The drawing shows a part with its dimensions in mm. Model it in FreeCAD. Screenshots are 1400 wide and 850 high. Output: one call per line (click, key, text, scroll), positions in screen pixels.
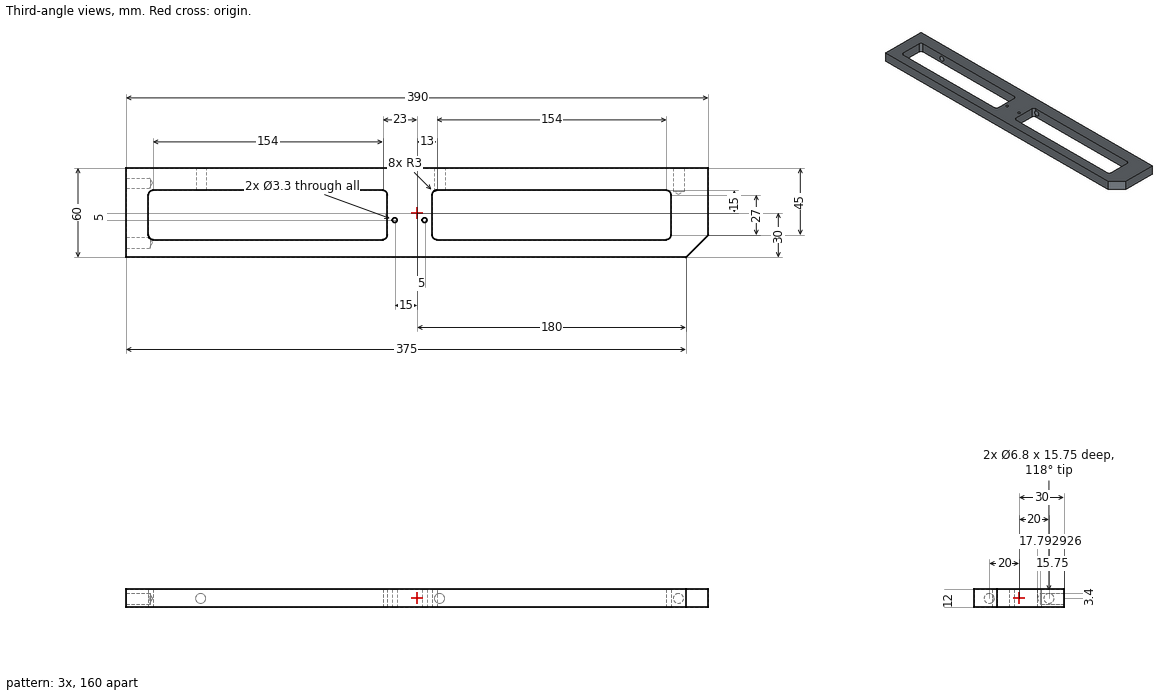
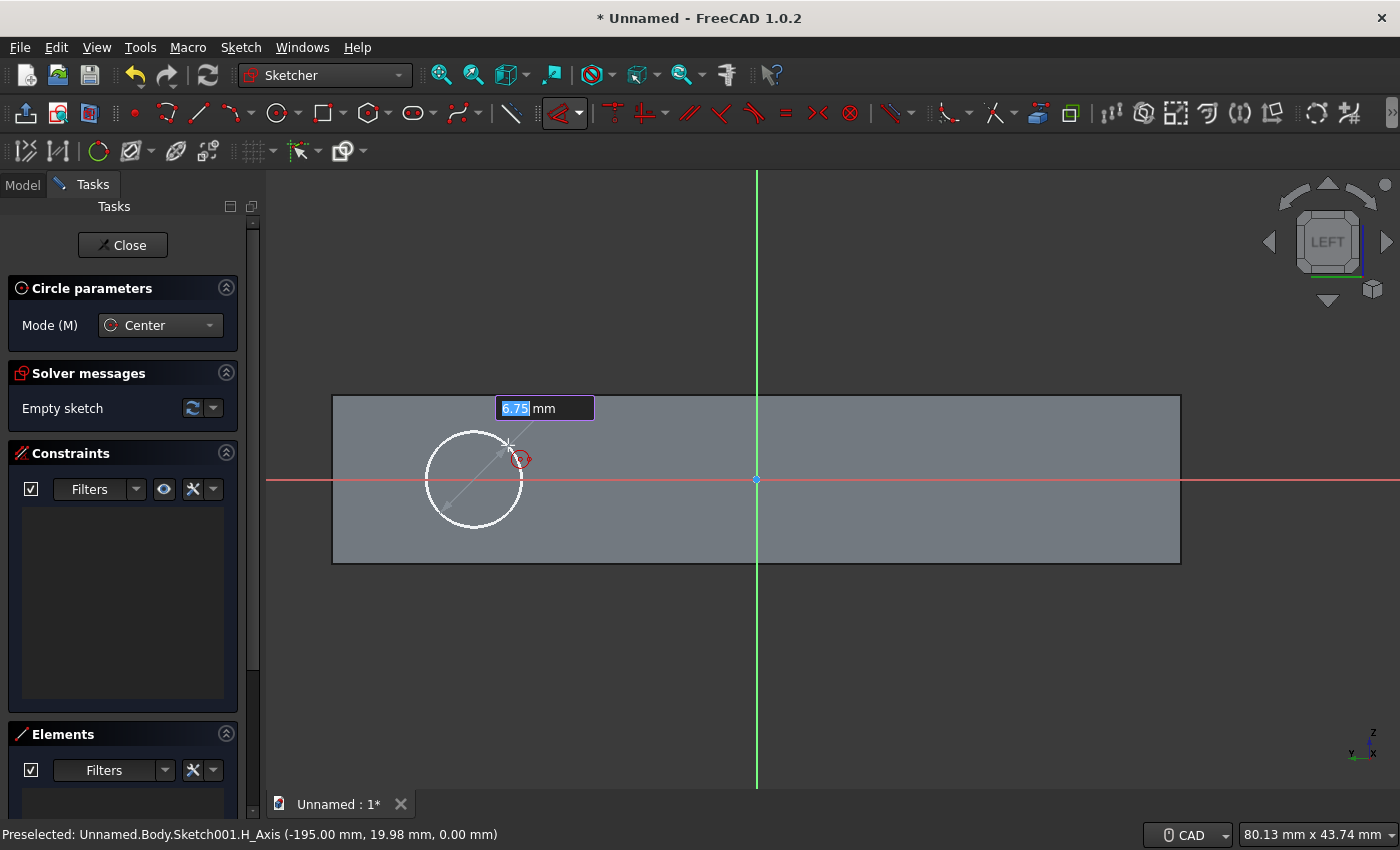
text(6.8)
key(Return)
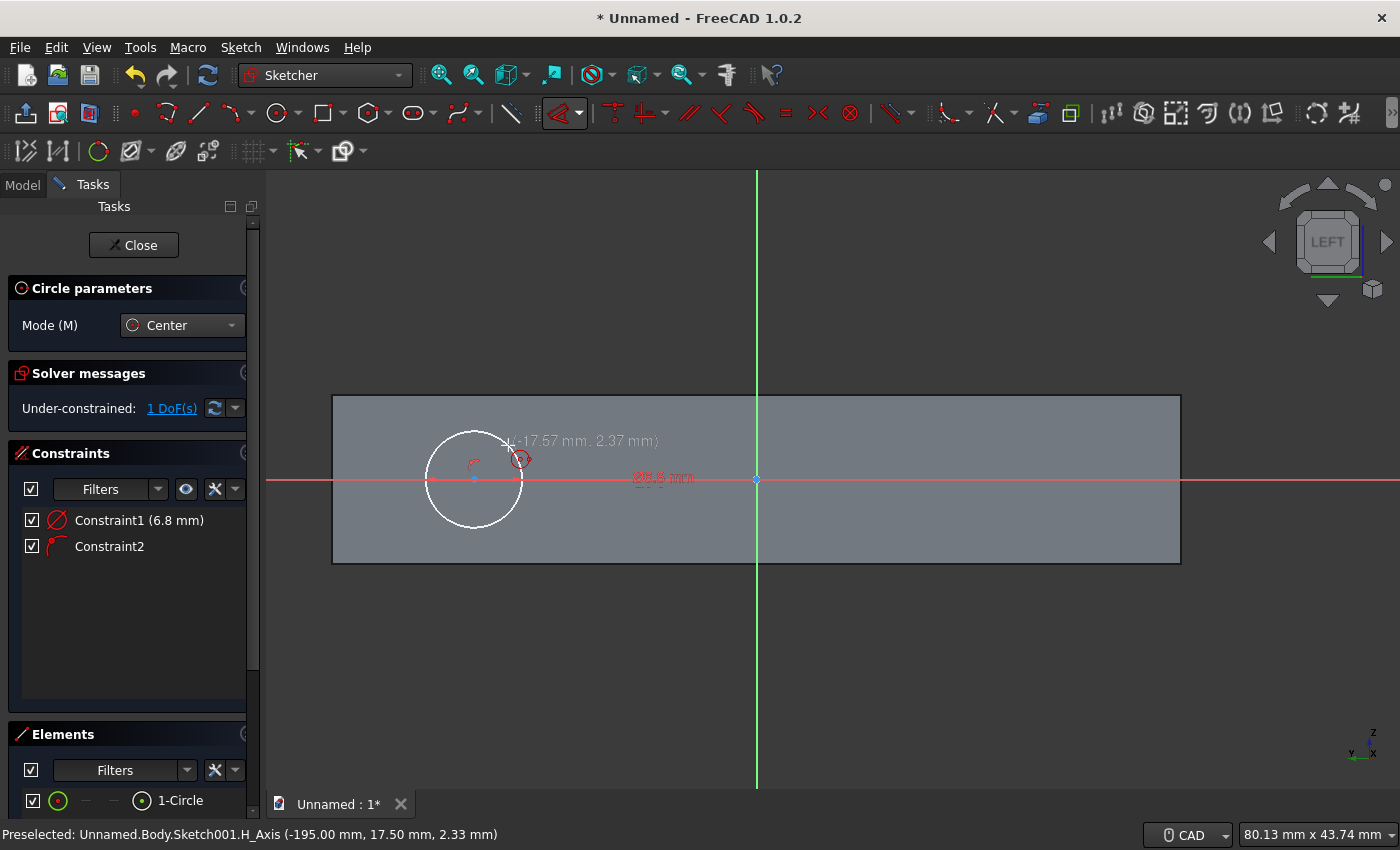
click(1040, 480)
move(1074, 445)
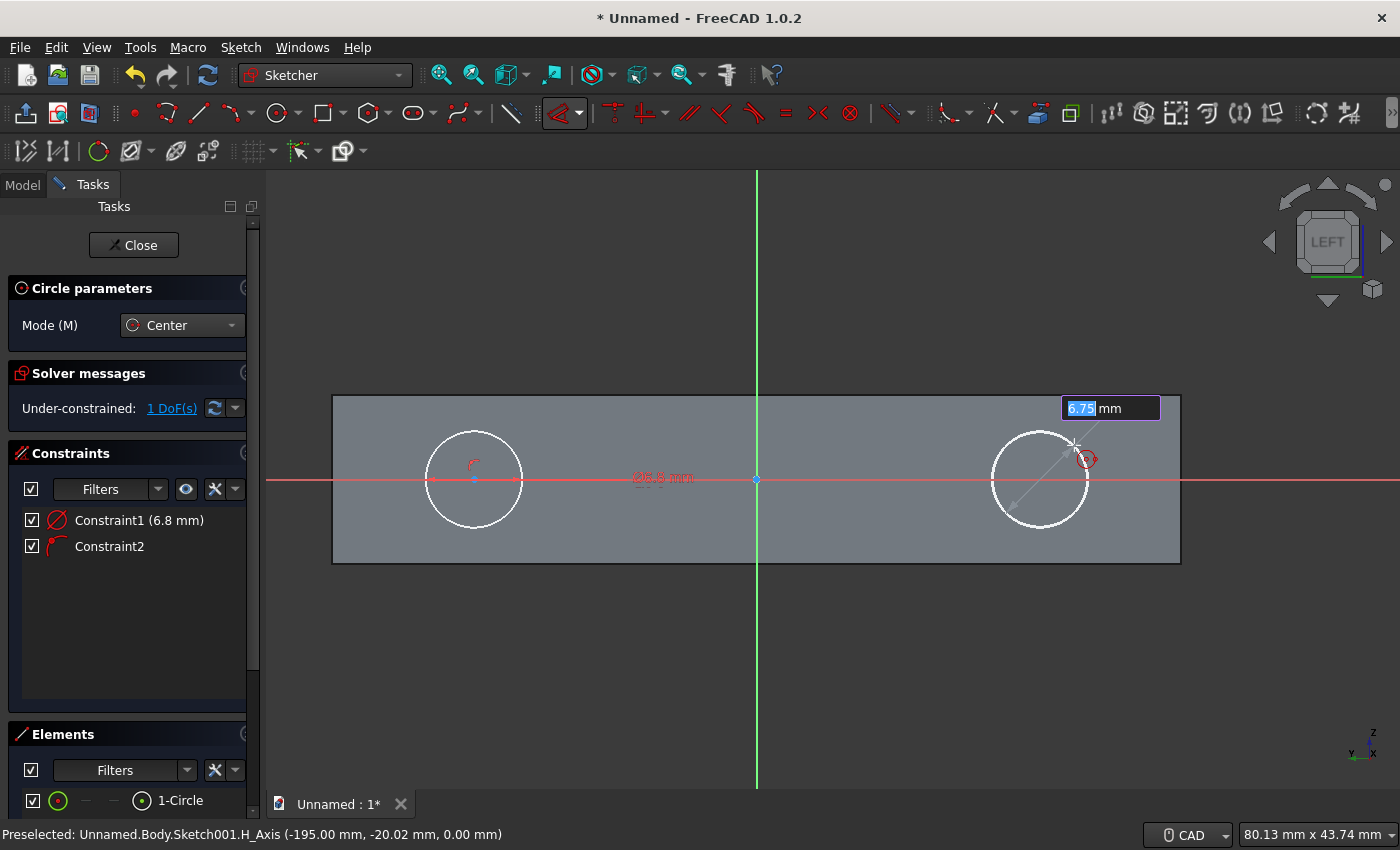
text(6.8)
key(Return)
key(Escape)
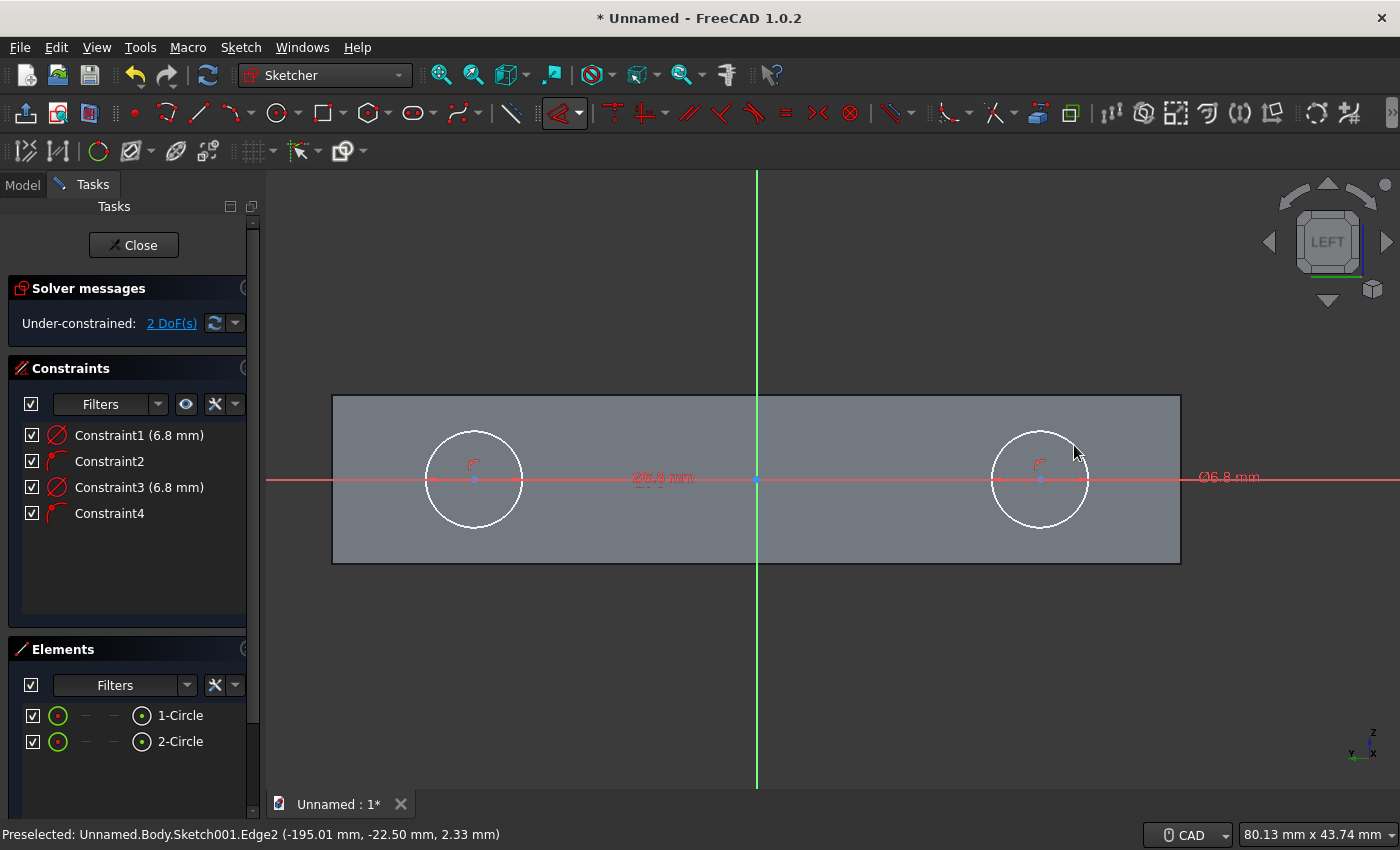
click(474, 480)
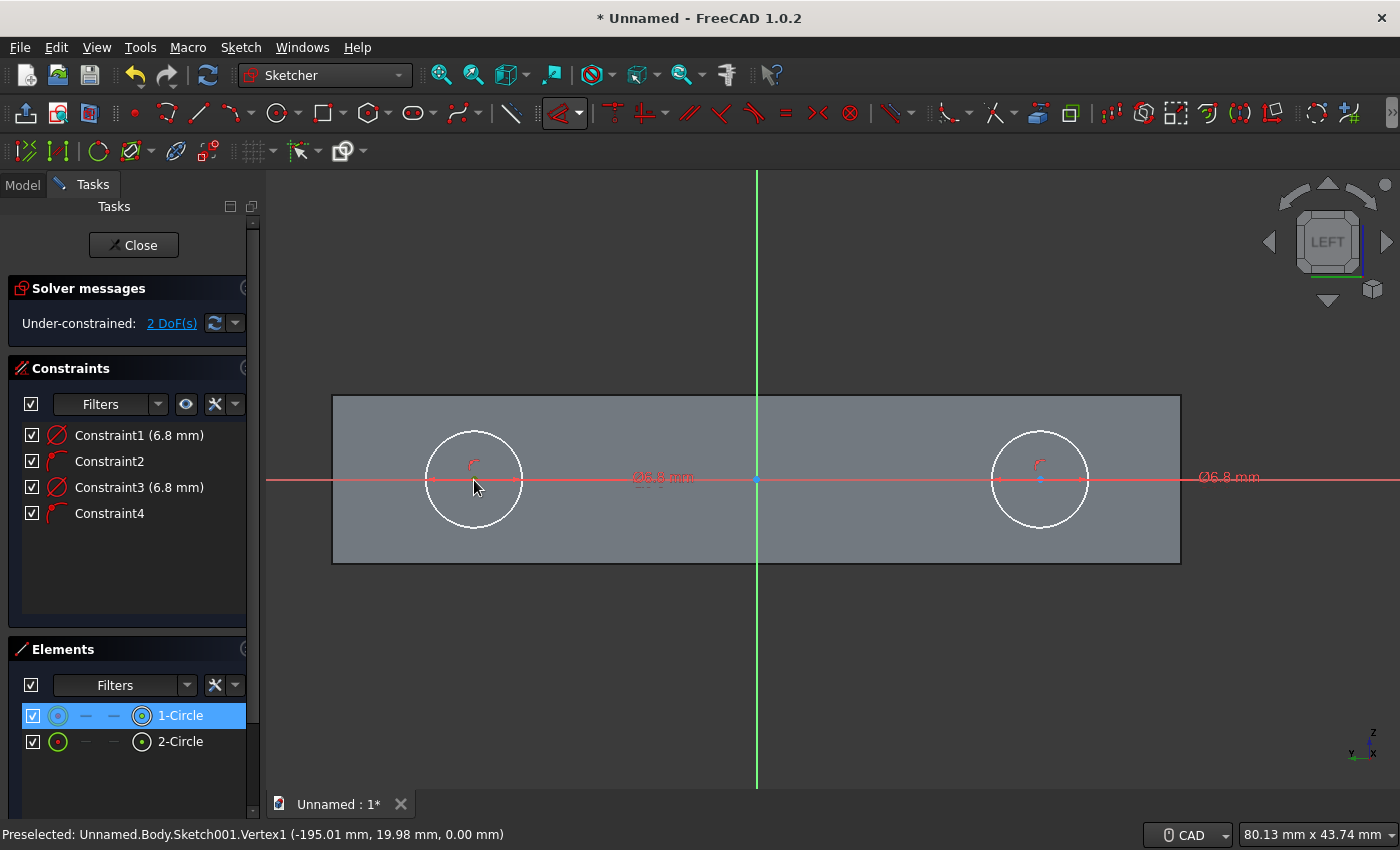
key(l)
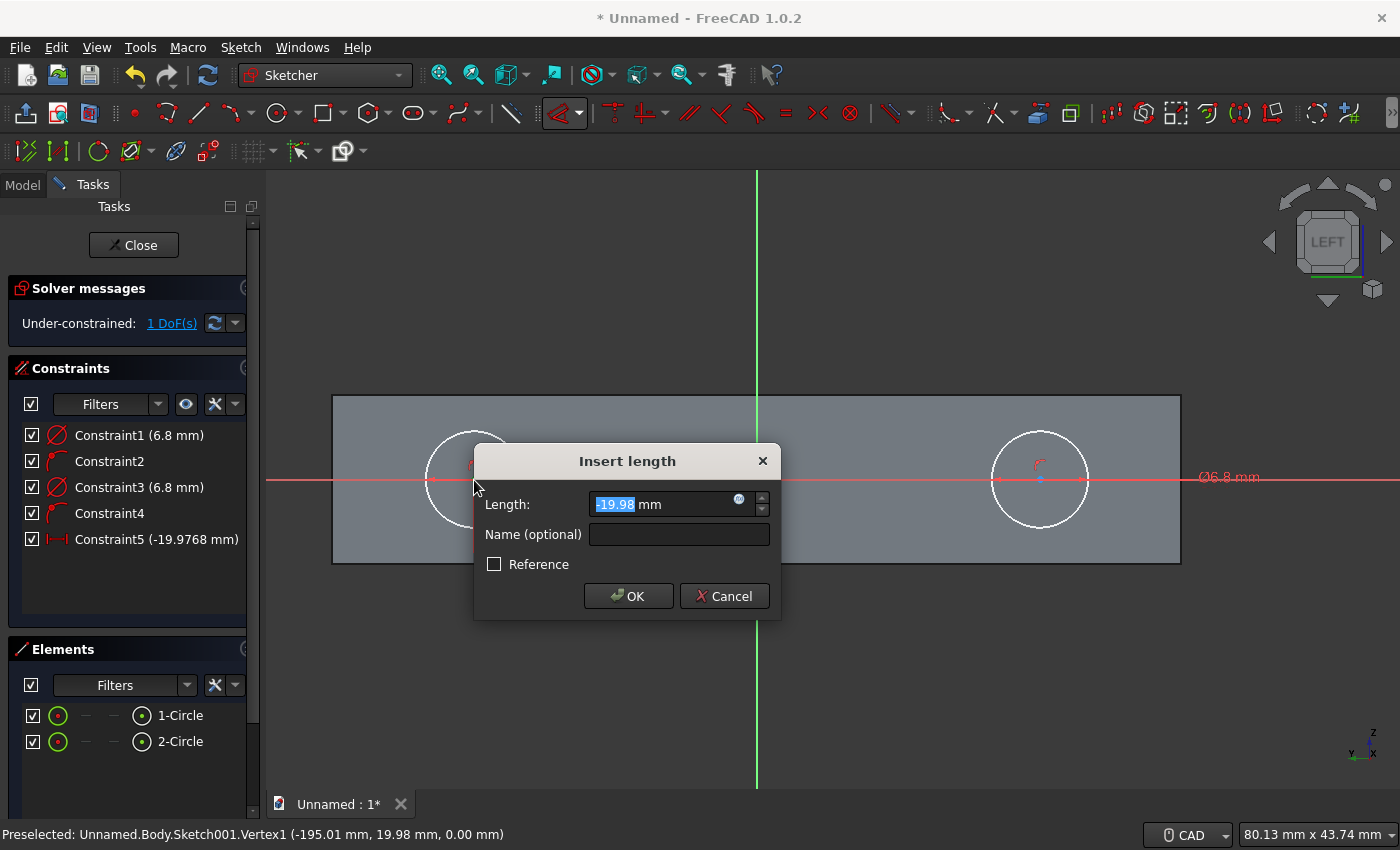
text(-20)
key(Return)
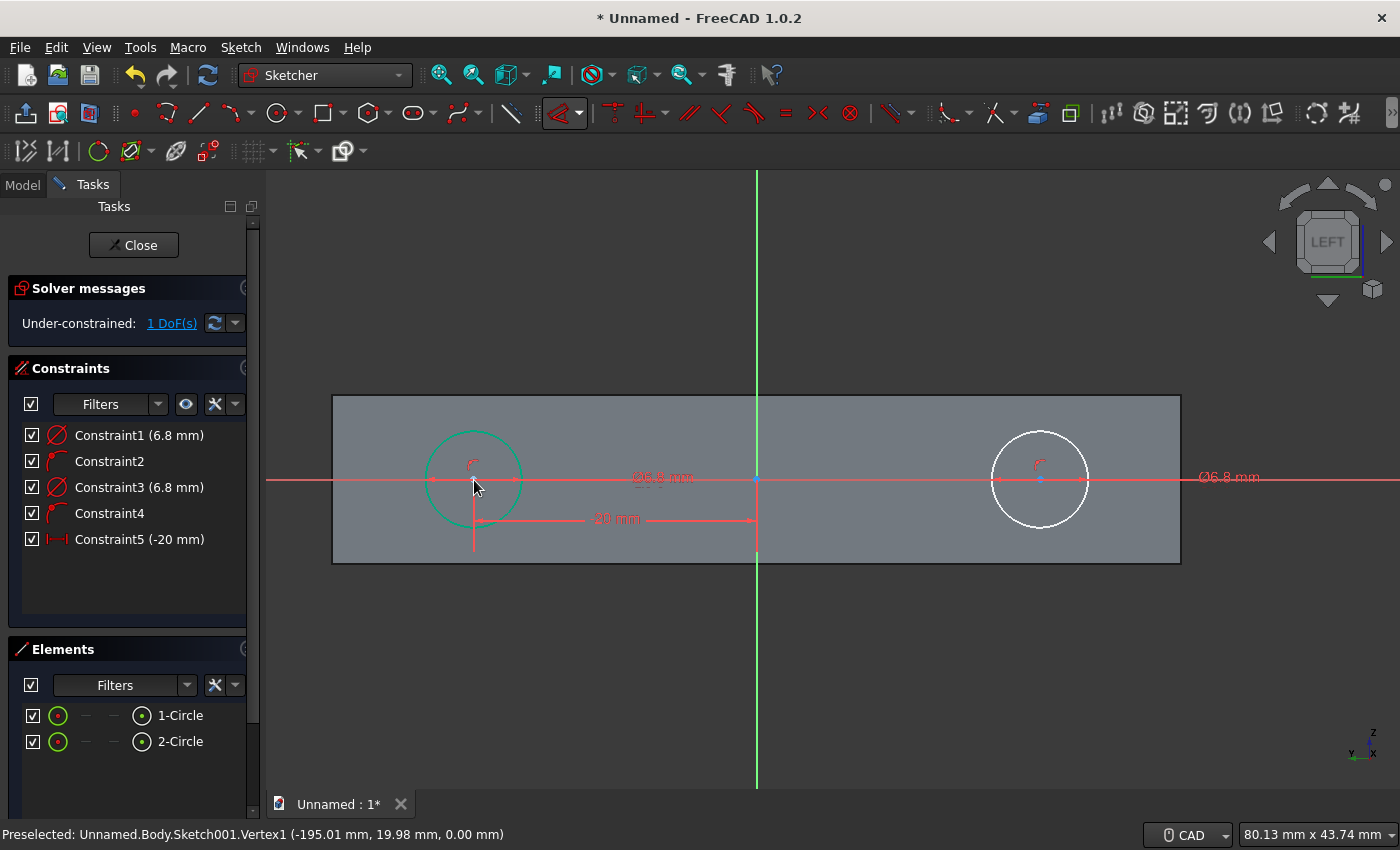
click(1040, 480)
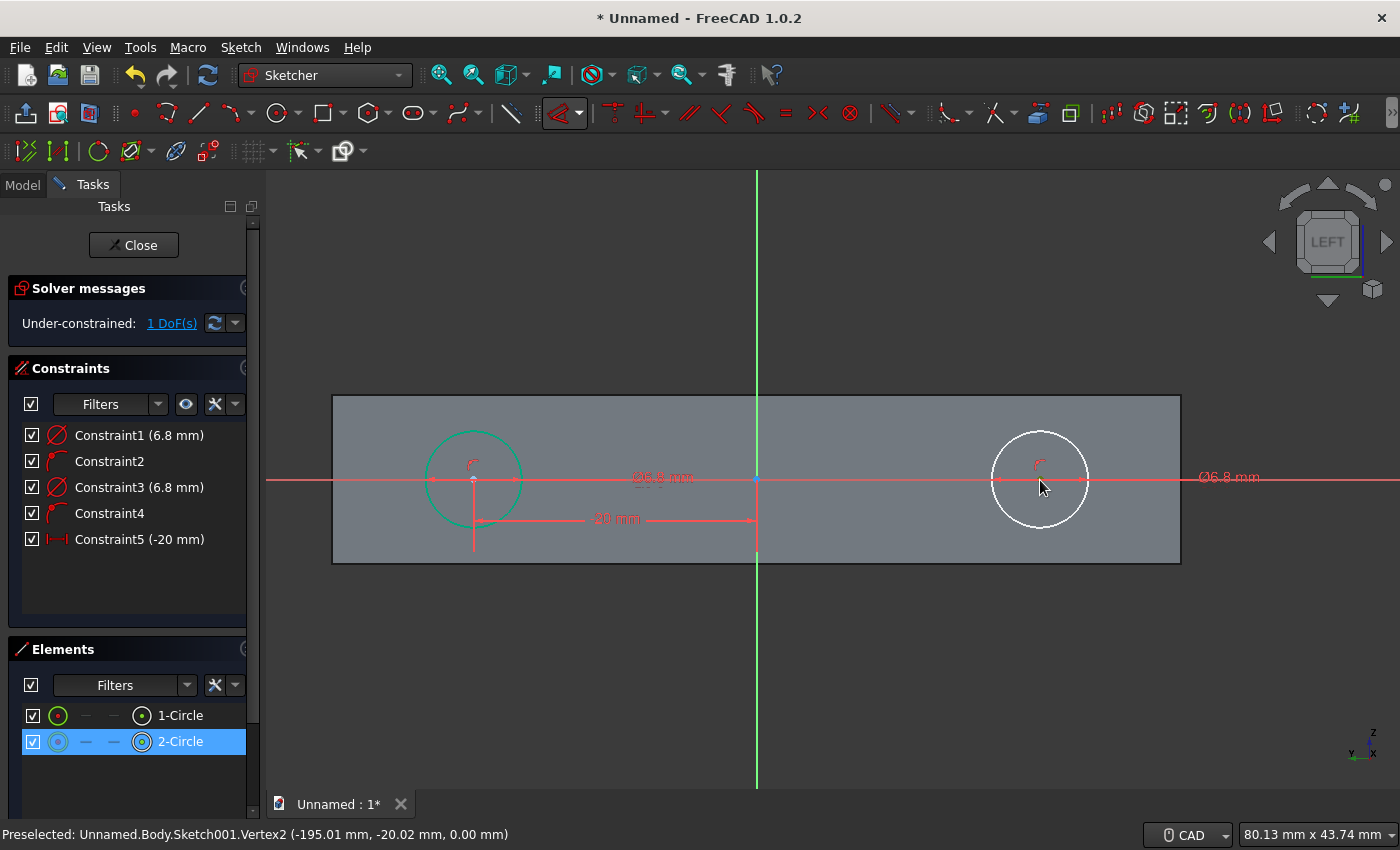
key(l)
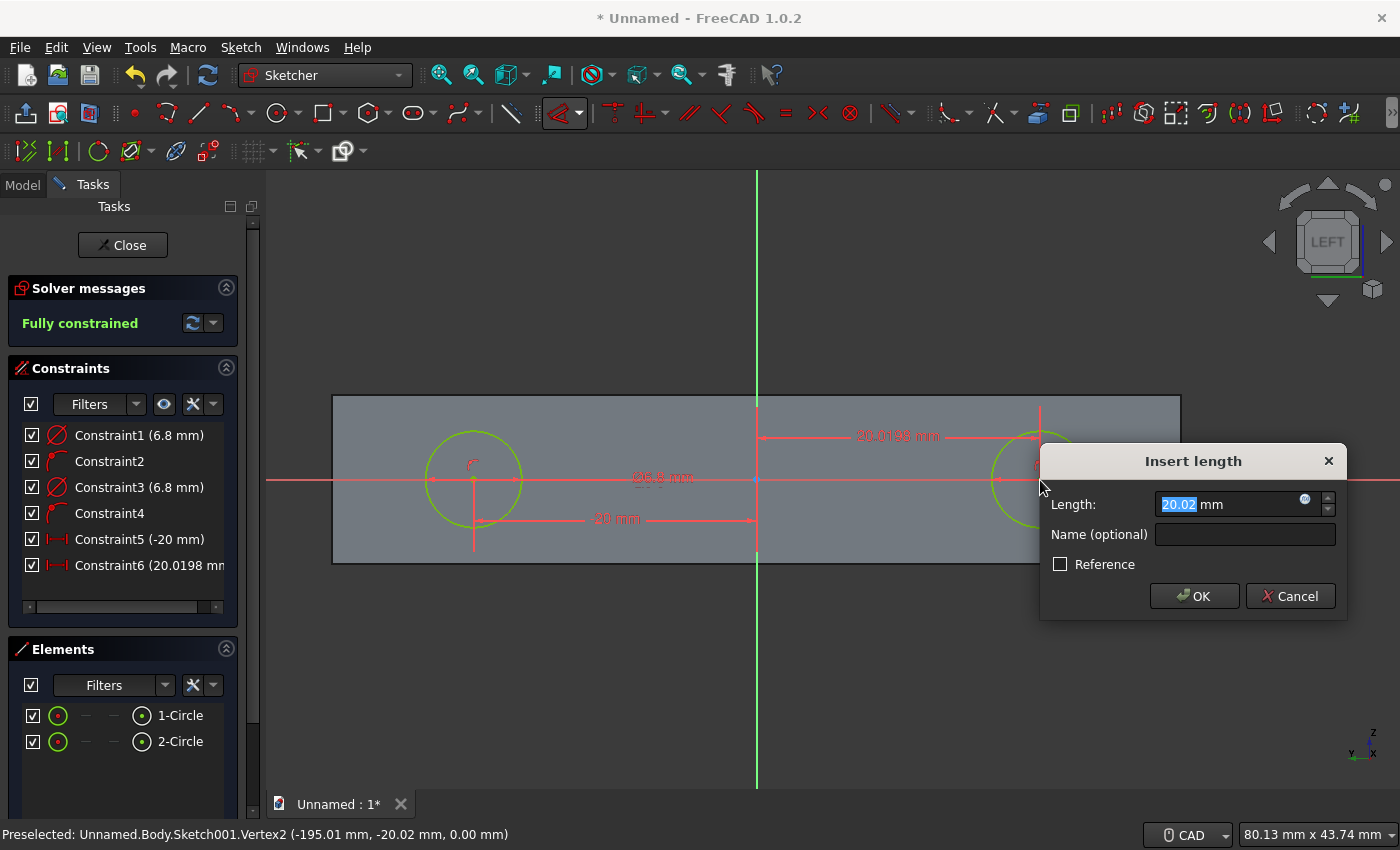
text(20)
key(Return)